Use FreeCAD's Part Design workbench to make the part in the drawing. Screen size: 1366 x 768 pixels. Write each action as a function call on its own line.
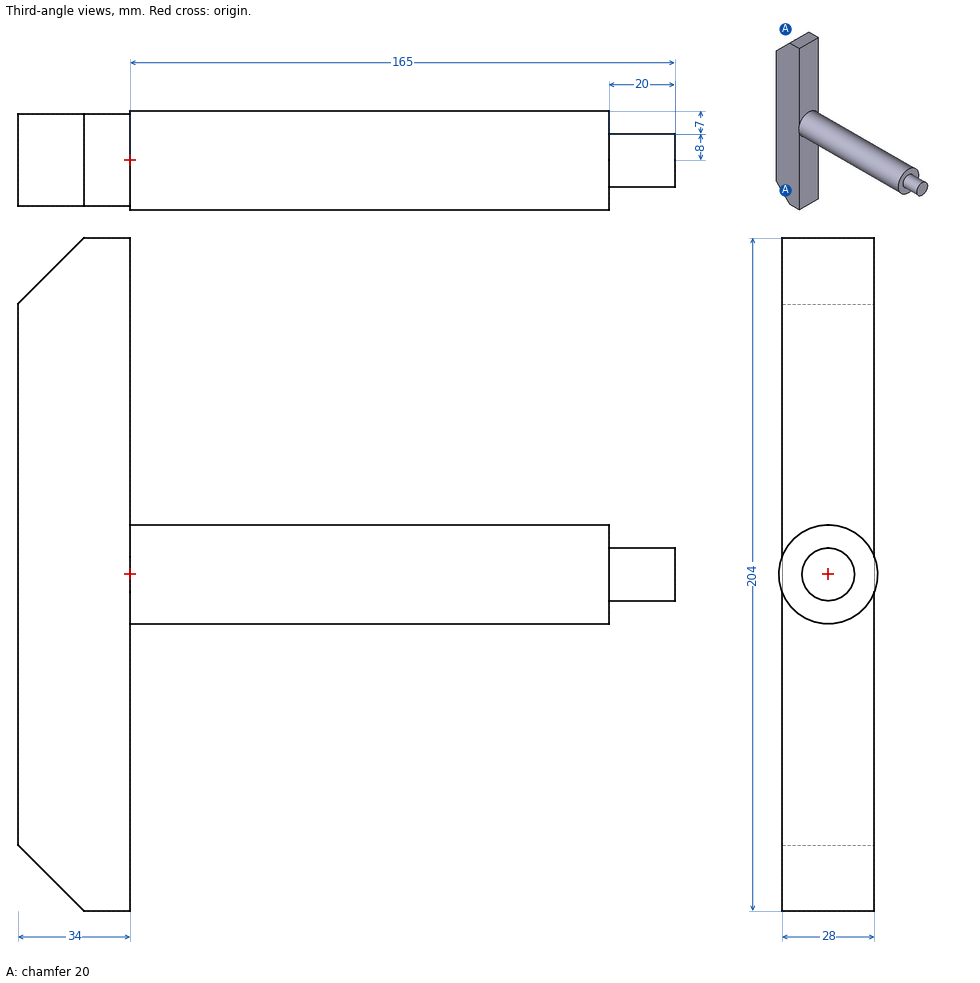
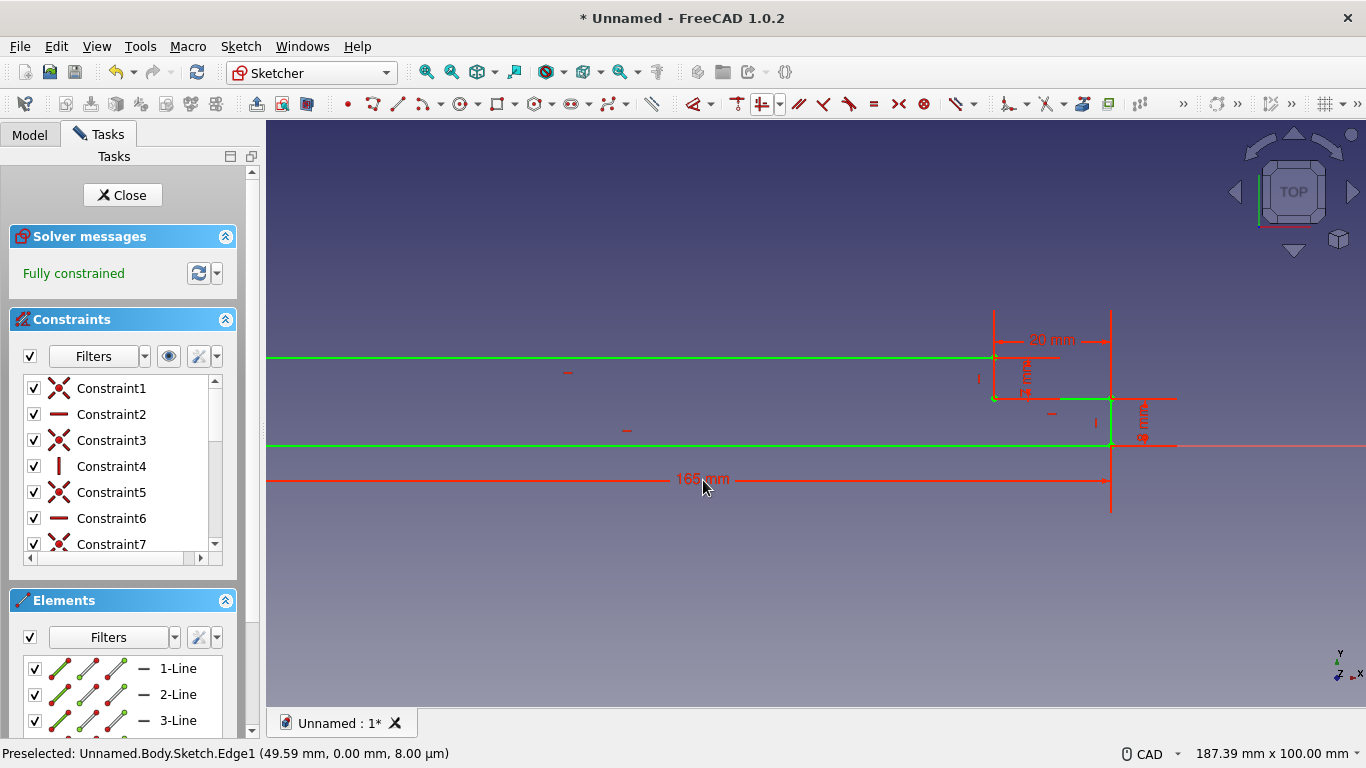
click(123, 195)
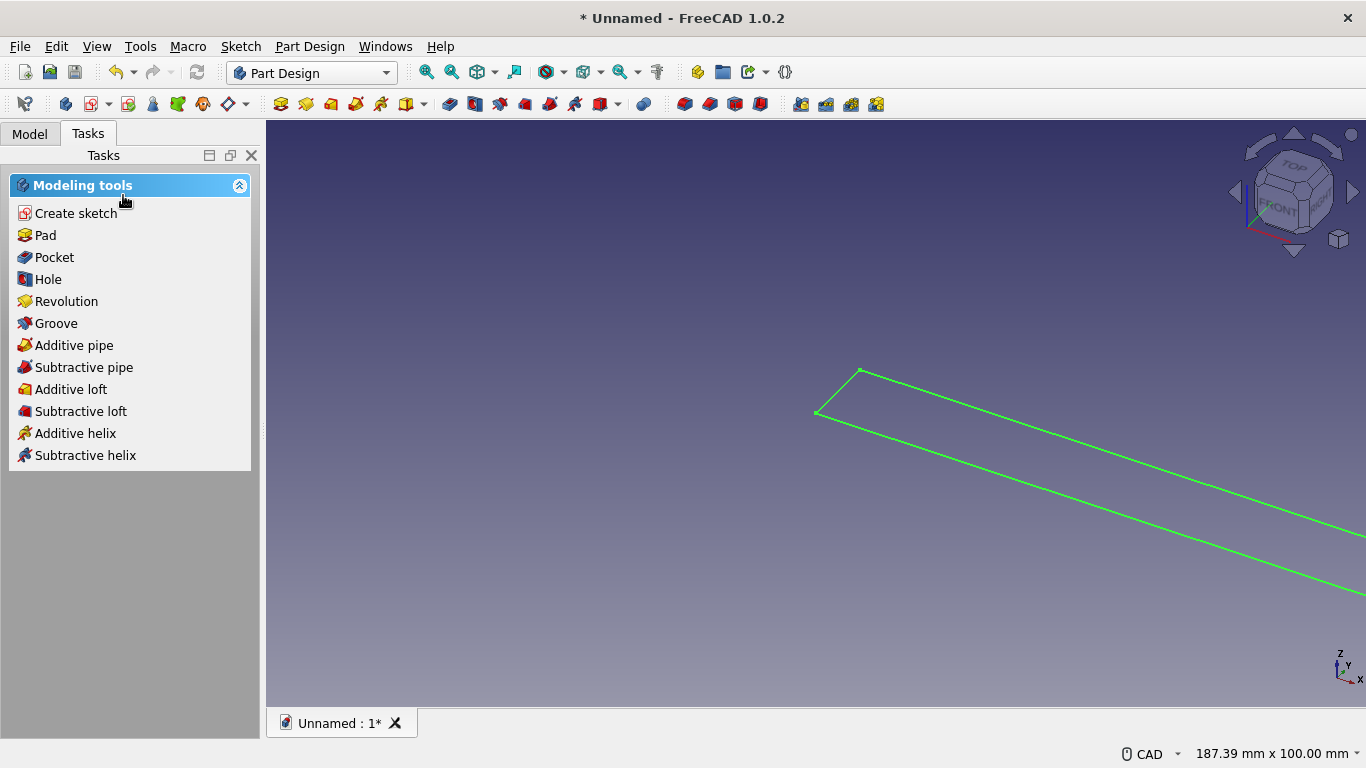
click(306, 104)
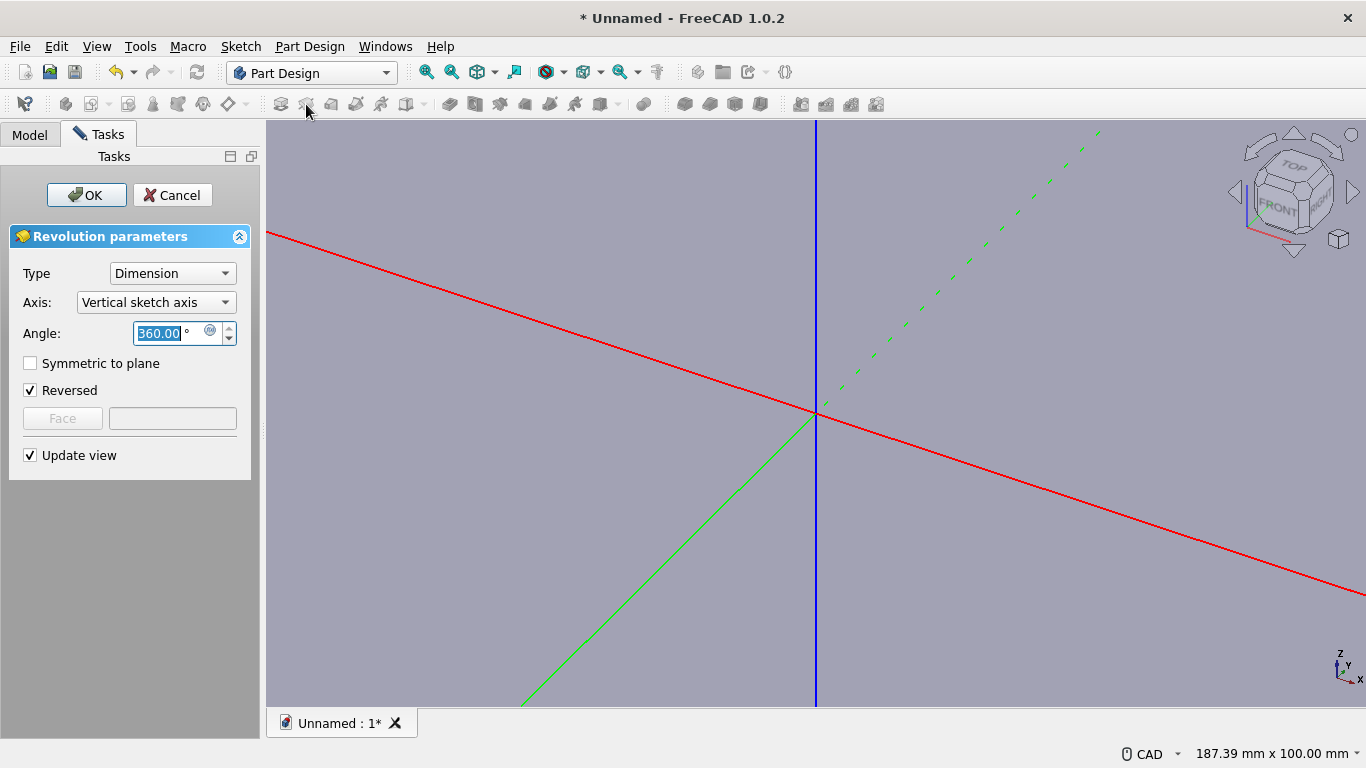
click(157, 302)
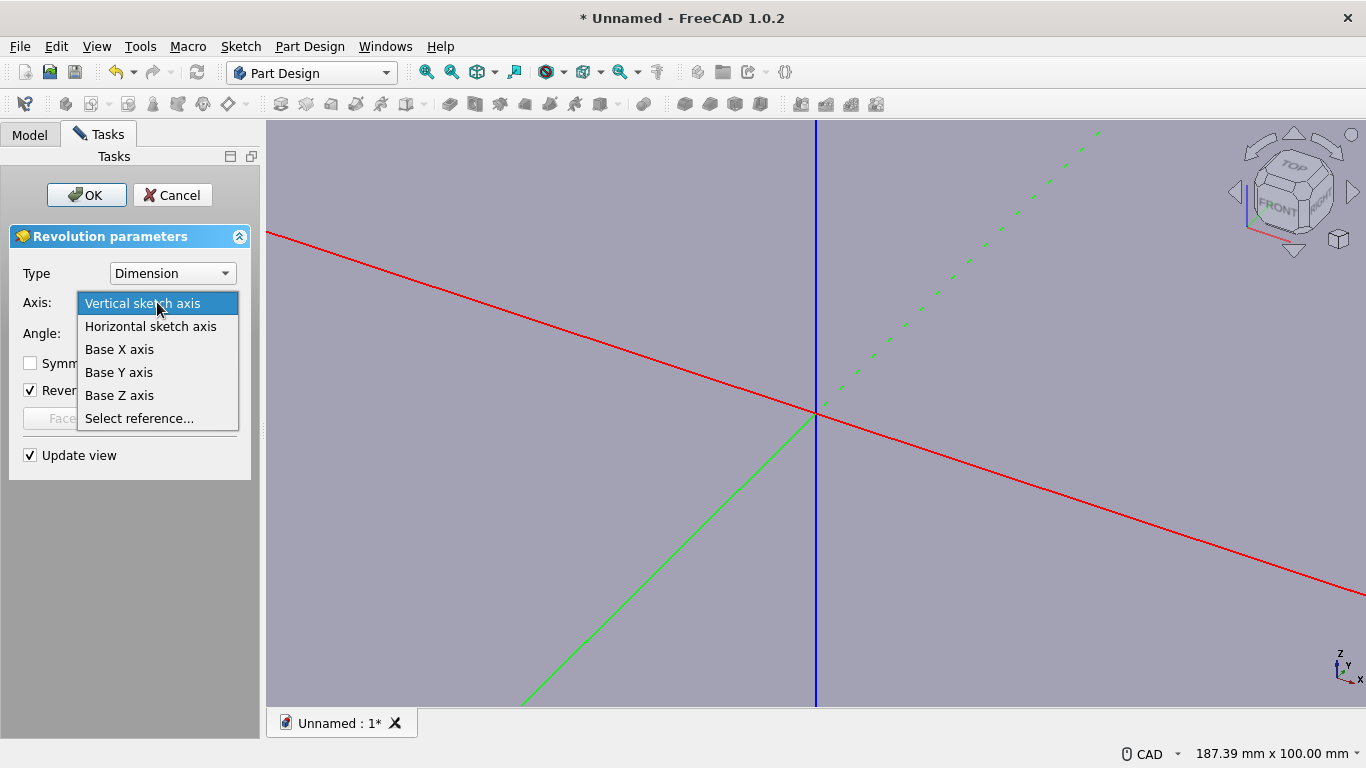
click(156, 326)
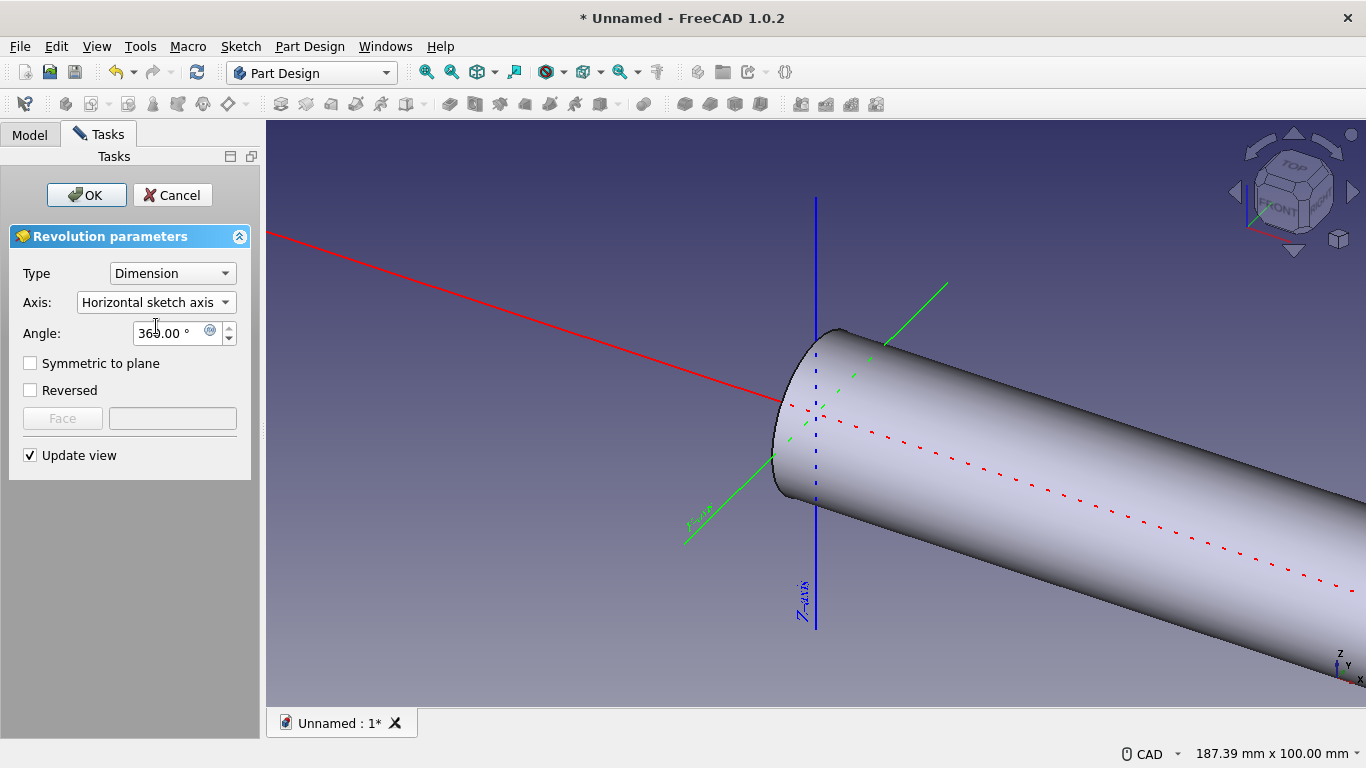
click(87, 195)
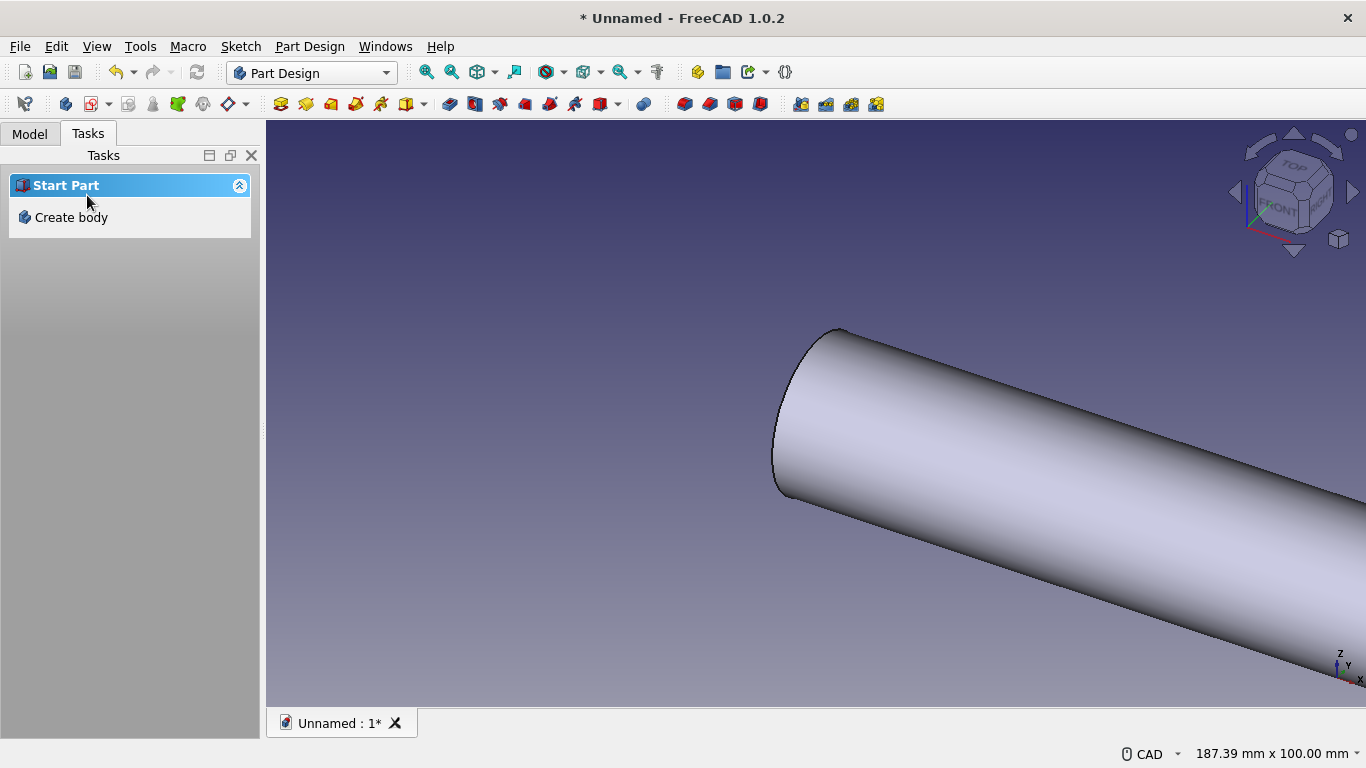
click(427, 72)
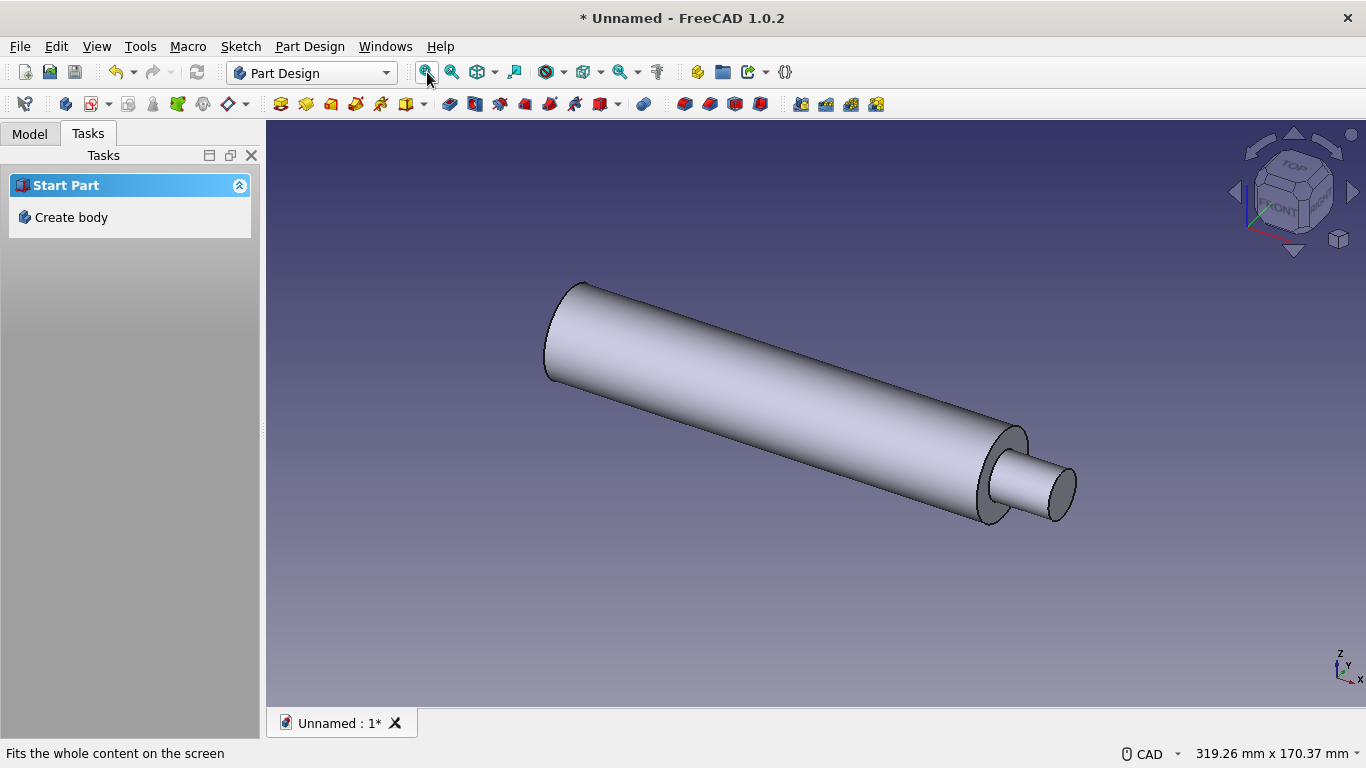
key(6)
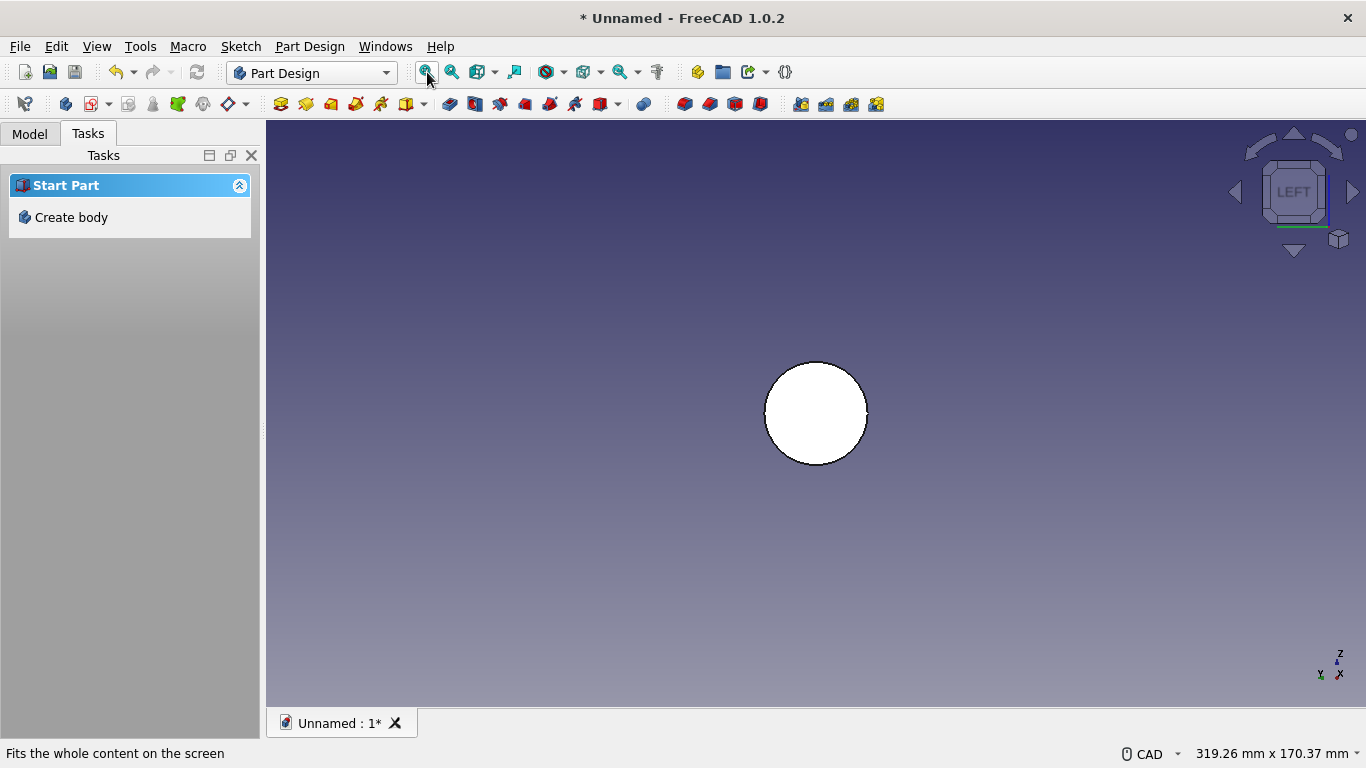
click(427, 72)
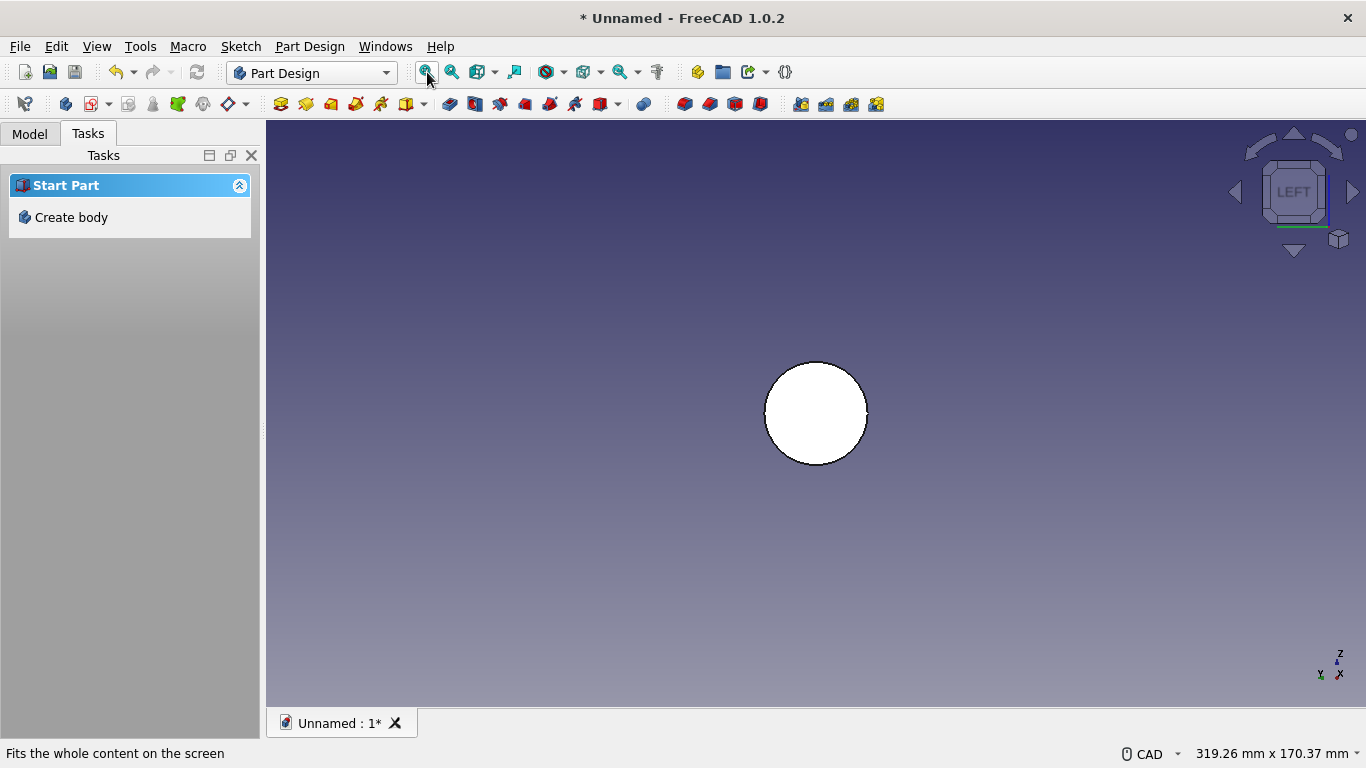
click(816, 412)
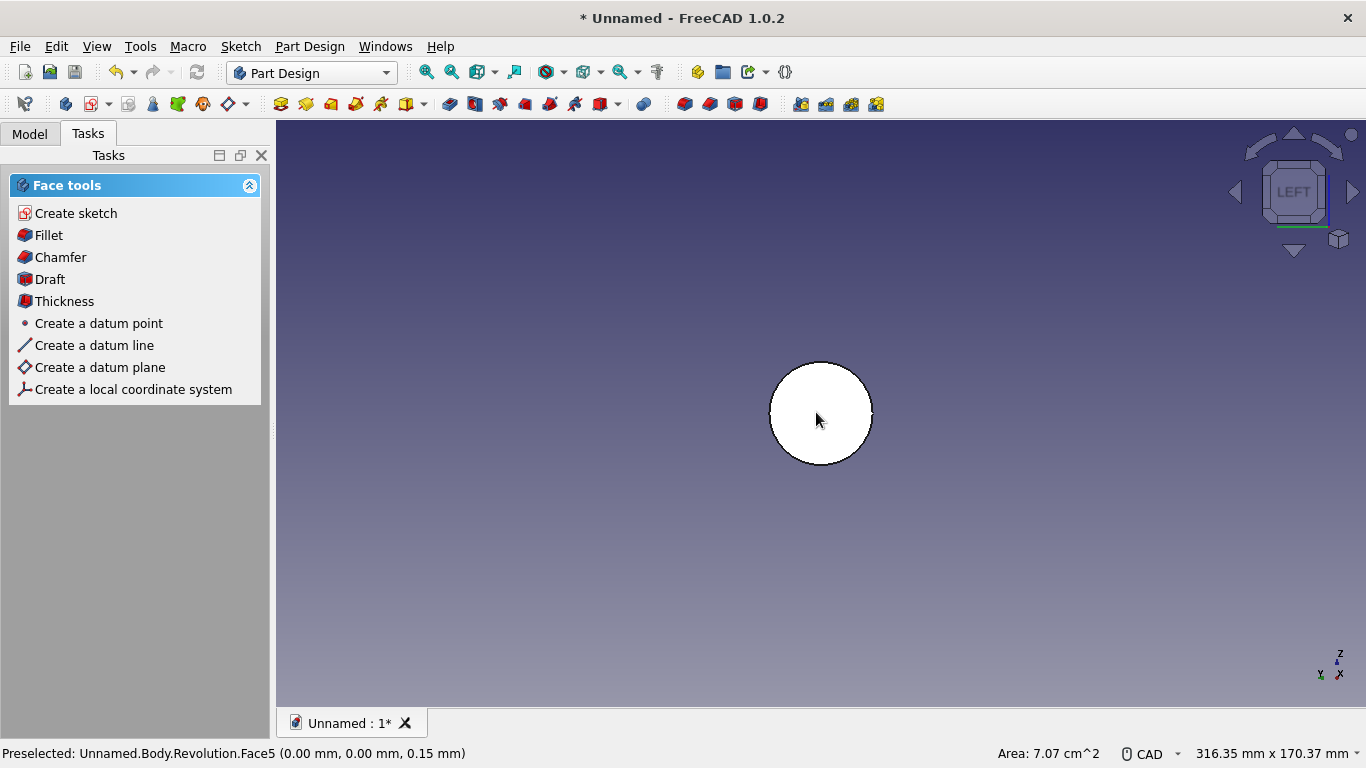
click(90, 104)